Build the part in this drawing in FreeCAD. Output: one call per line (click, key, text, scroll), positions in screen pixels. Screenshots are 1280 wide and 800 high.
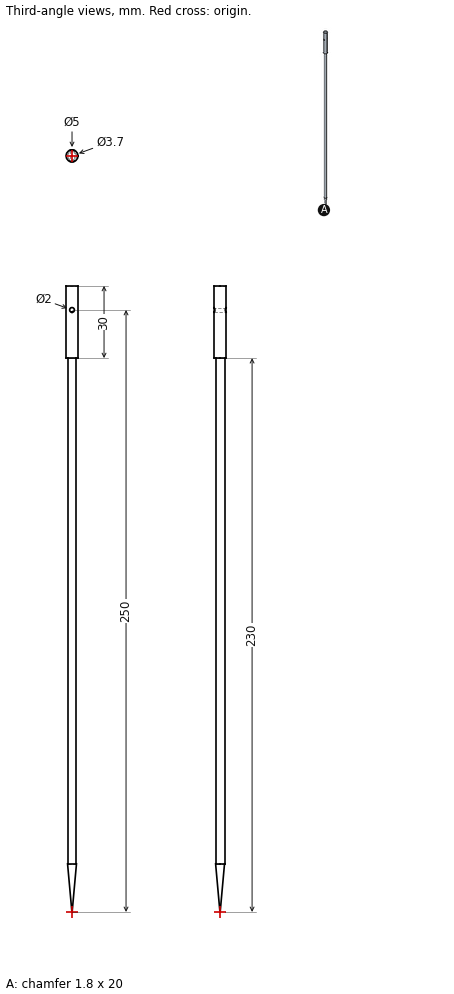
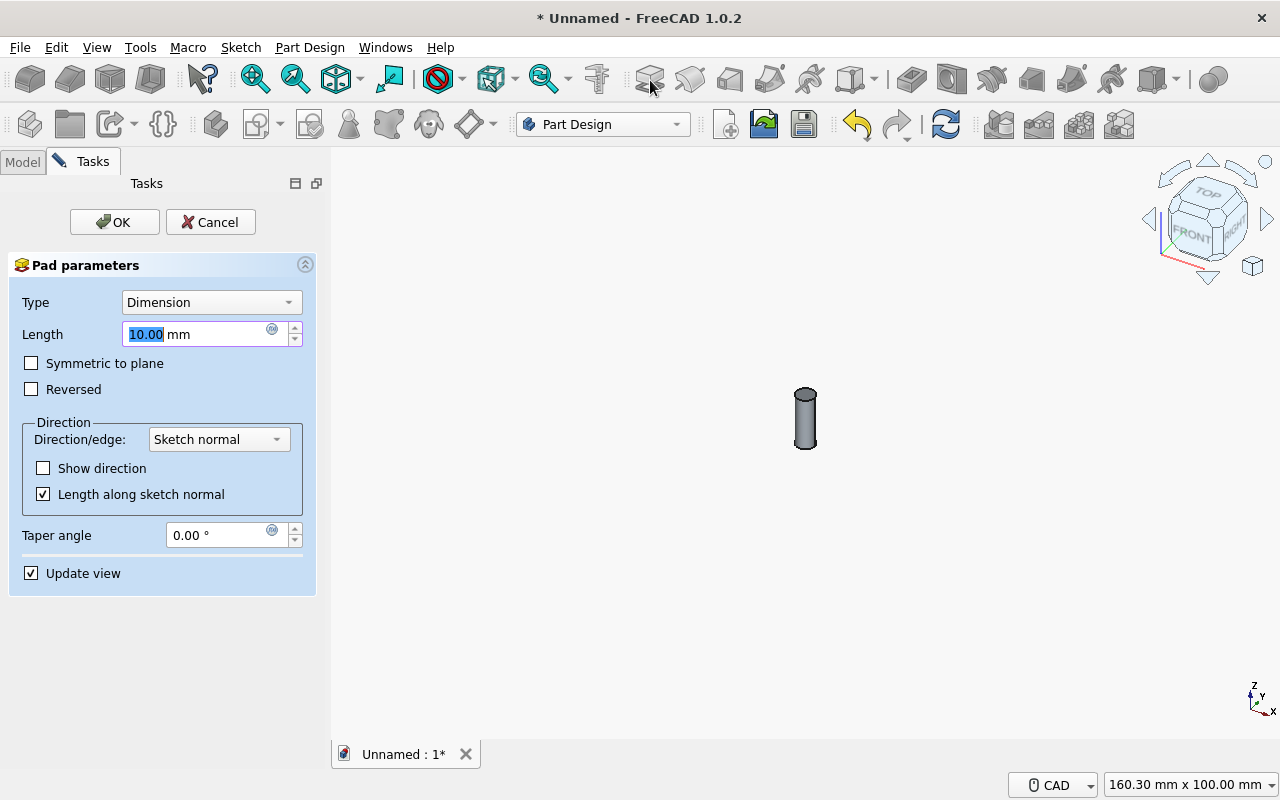
text(230)
key(Tab)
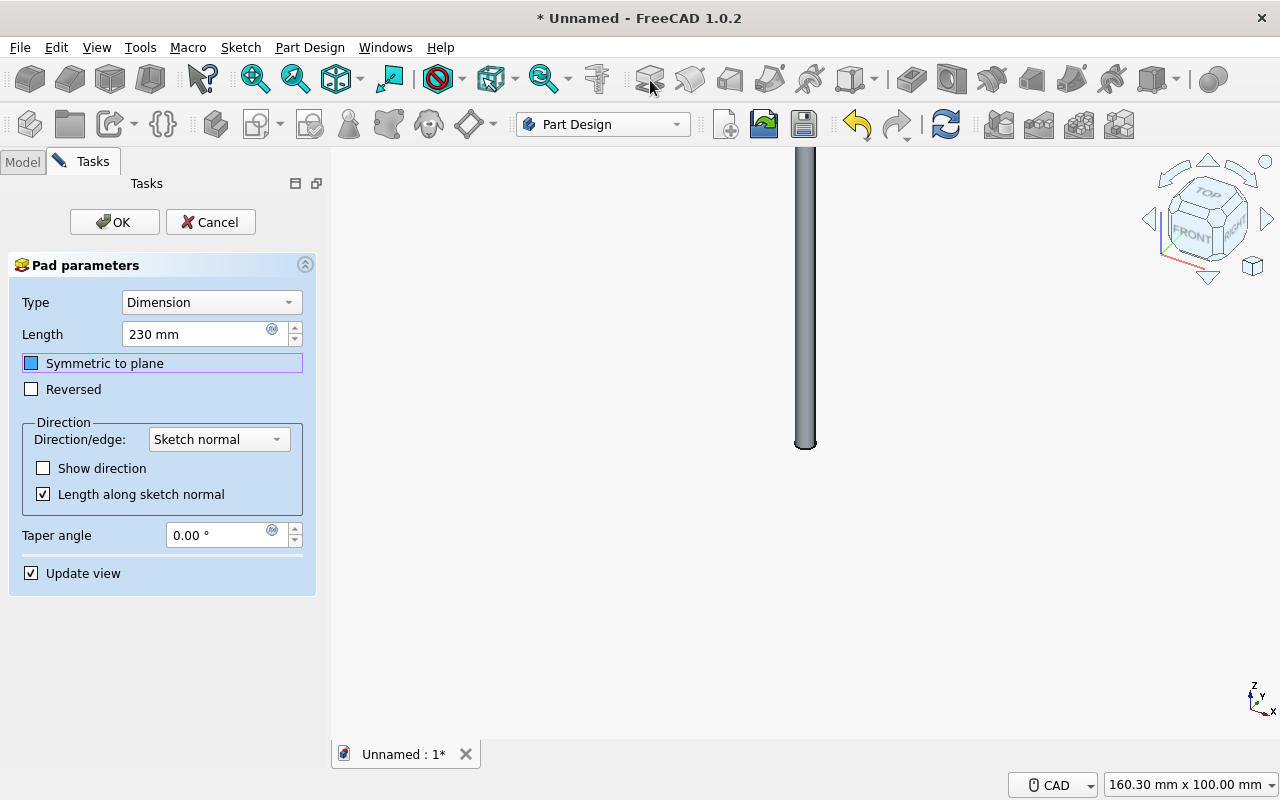
click(115, 222)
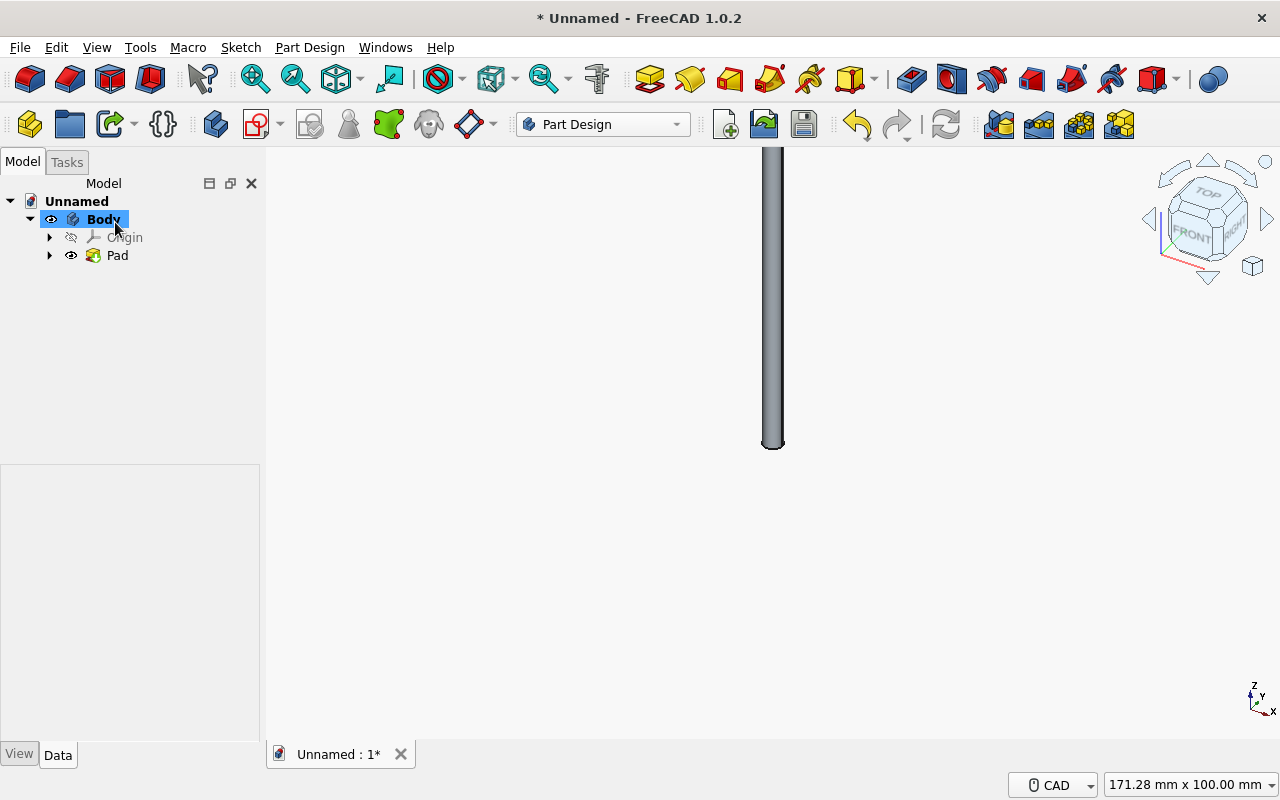
click(256, 80)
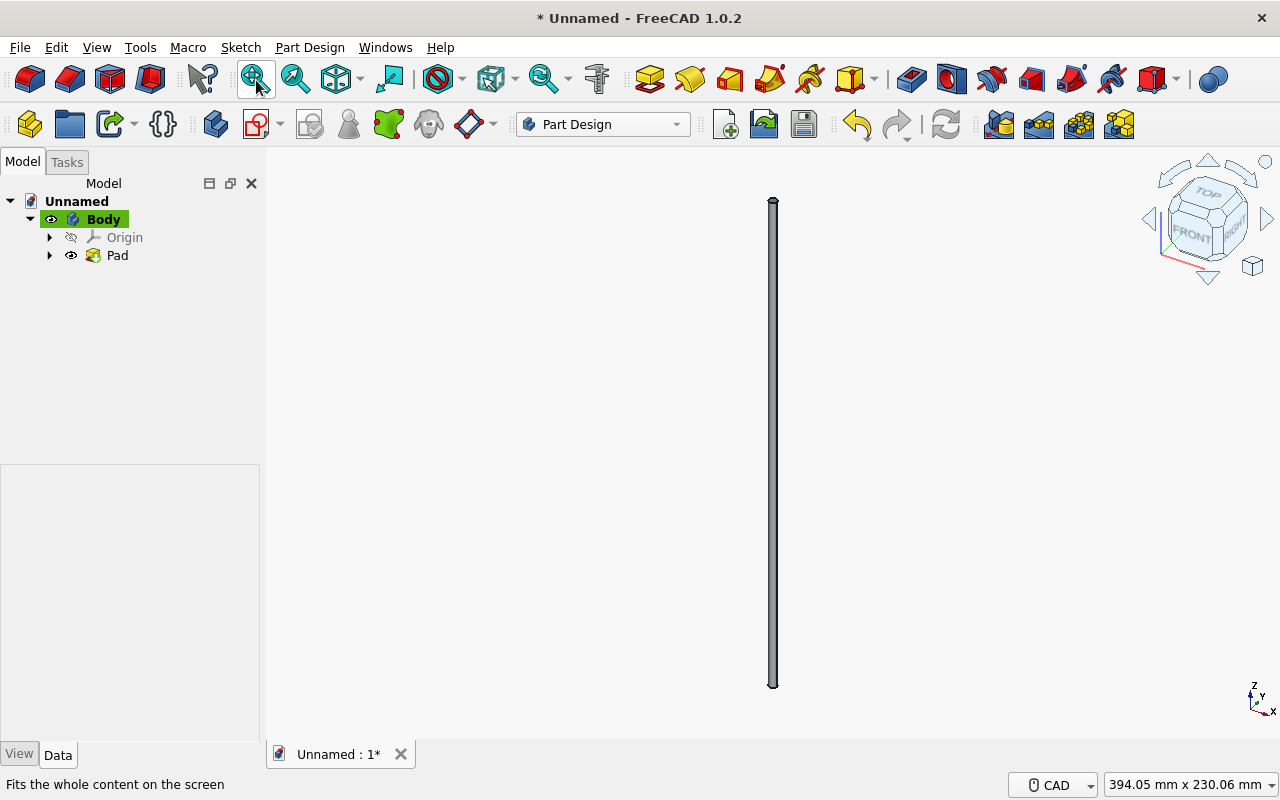
scroll(773, 200, up, 5)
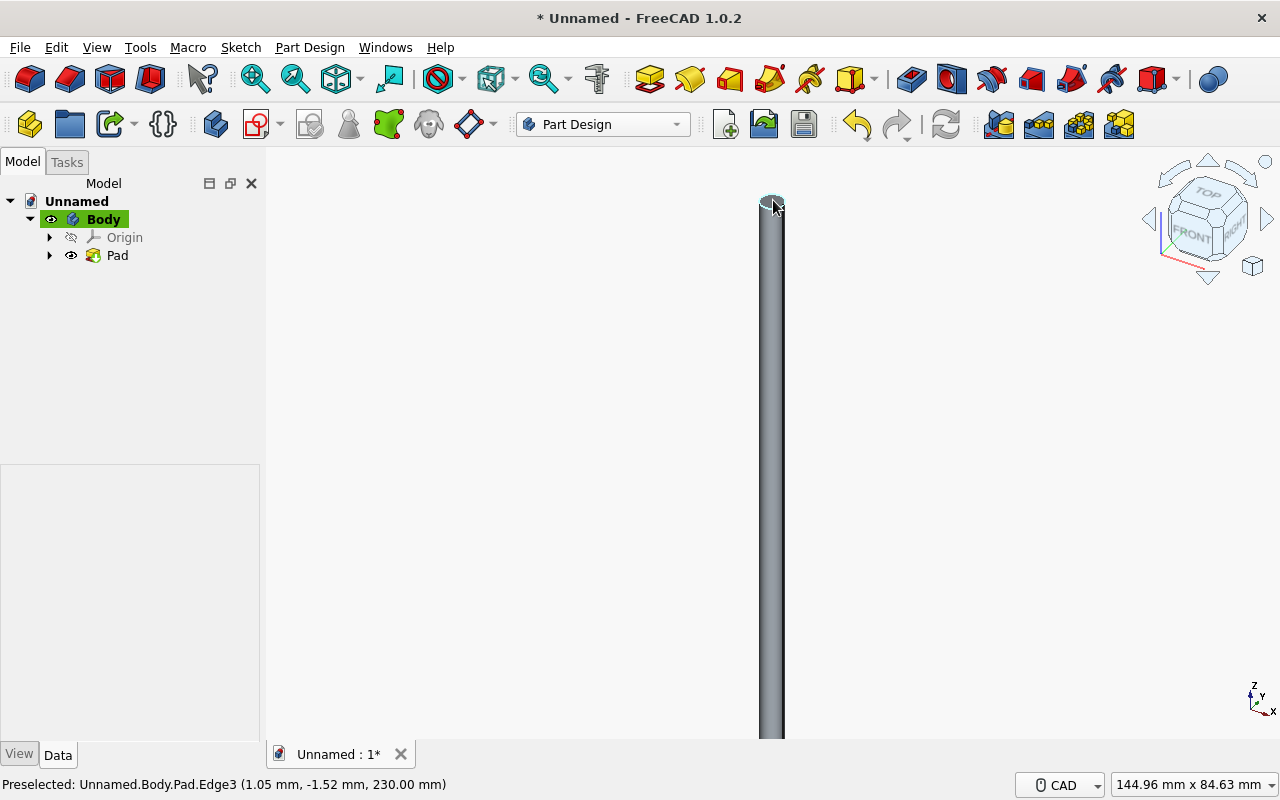
click(774, 199)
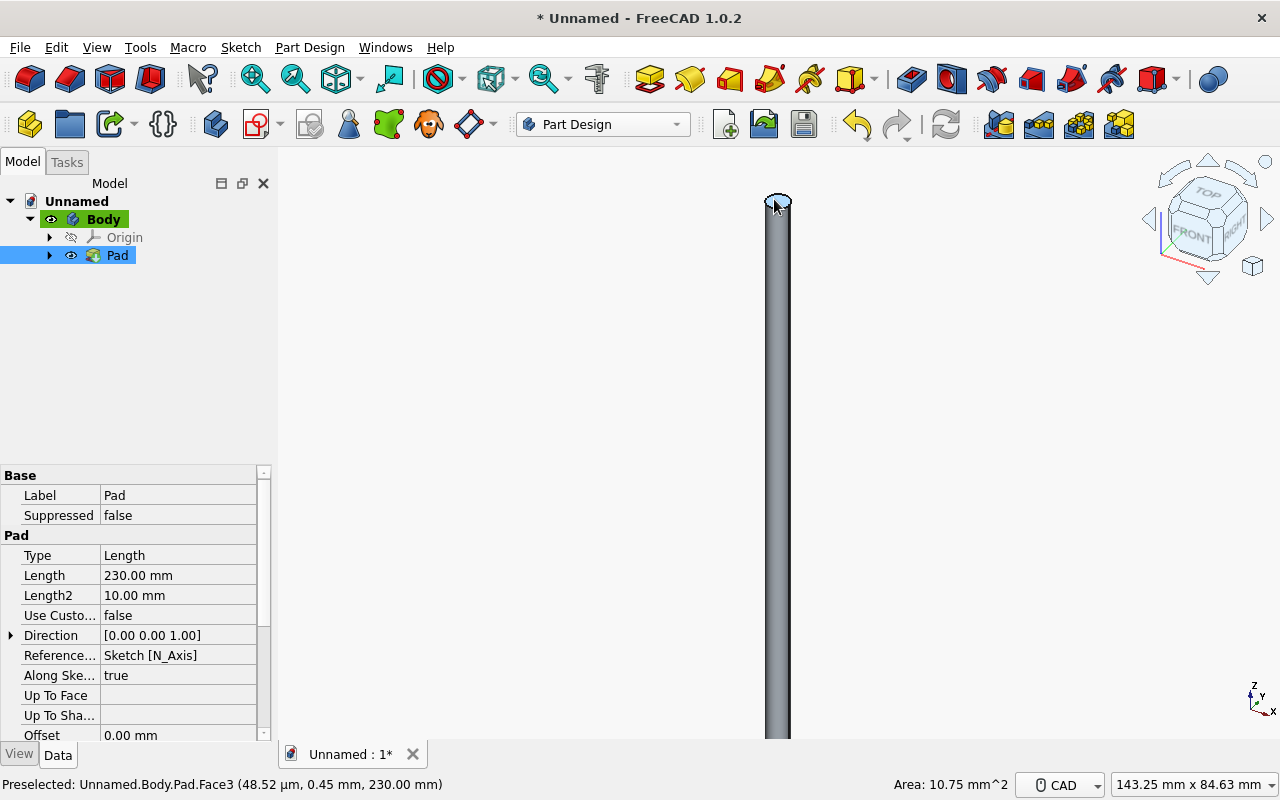
click(256, 124)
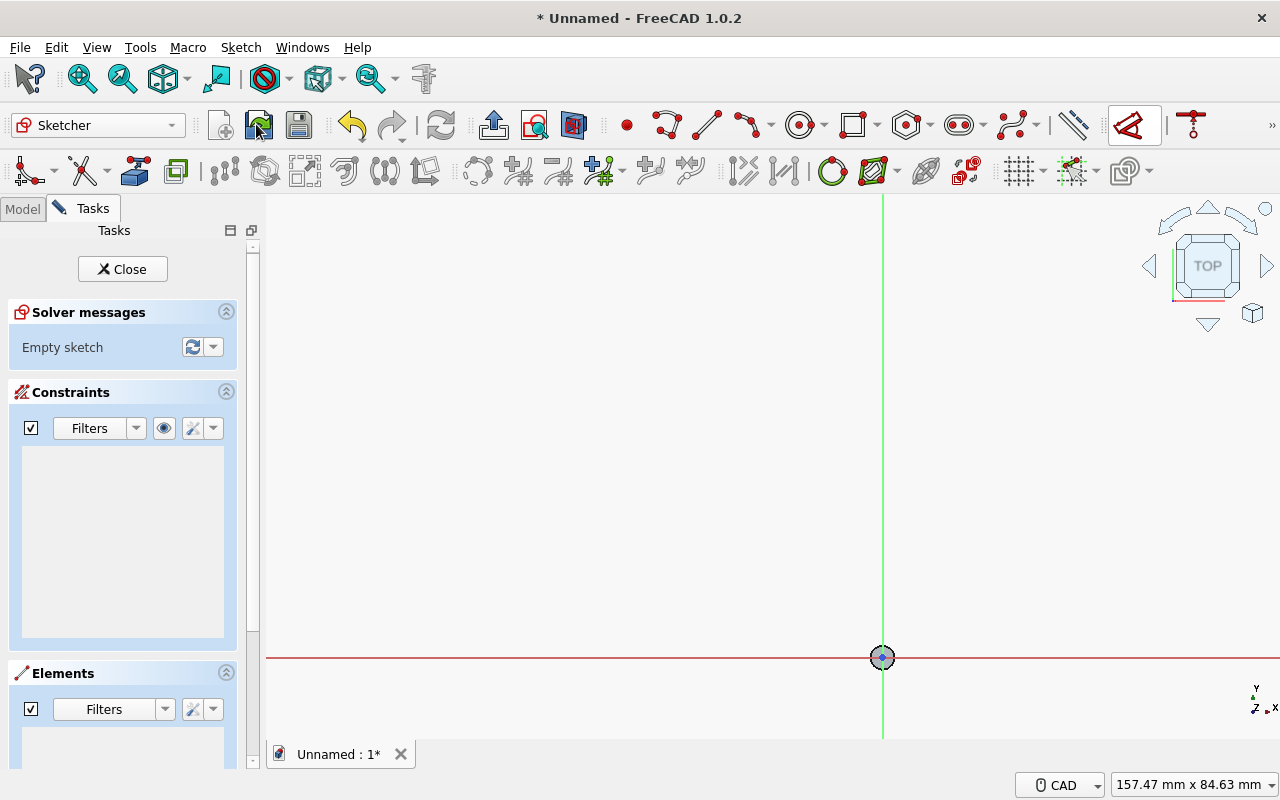
scroll(900, 677, up, 12)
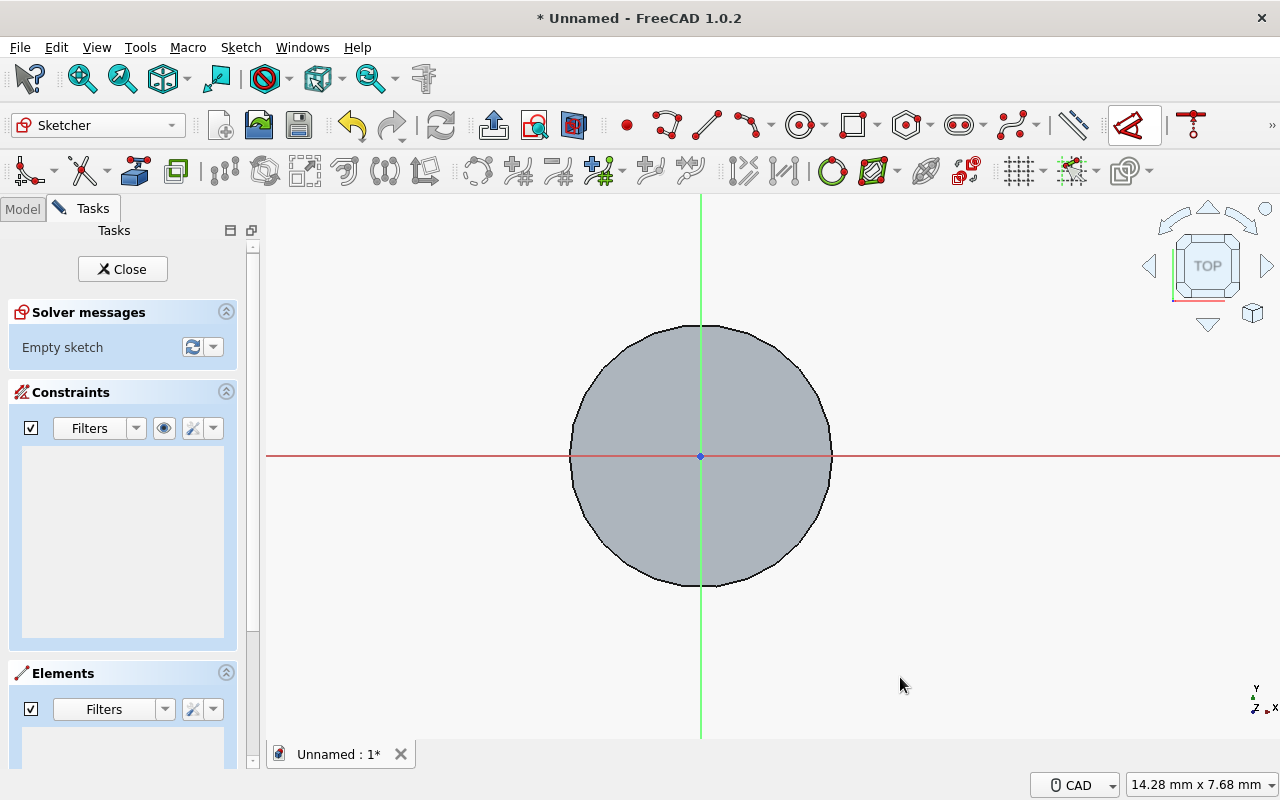
click(800, 126)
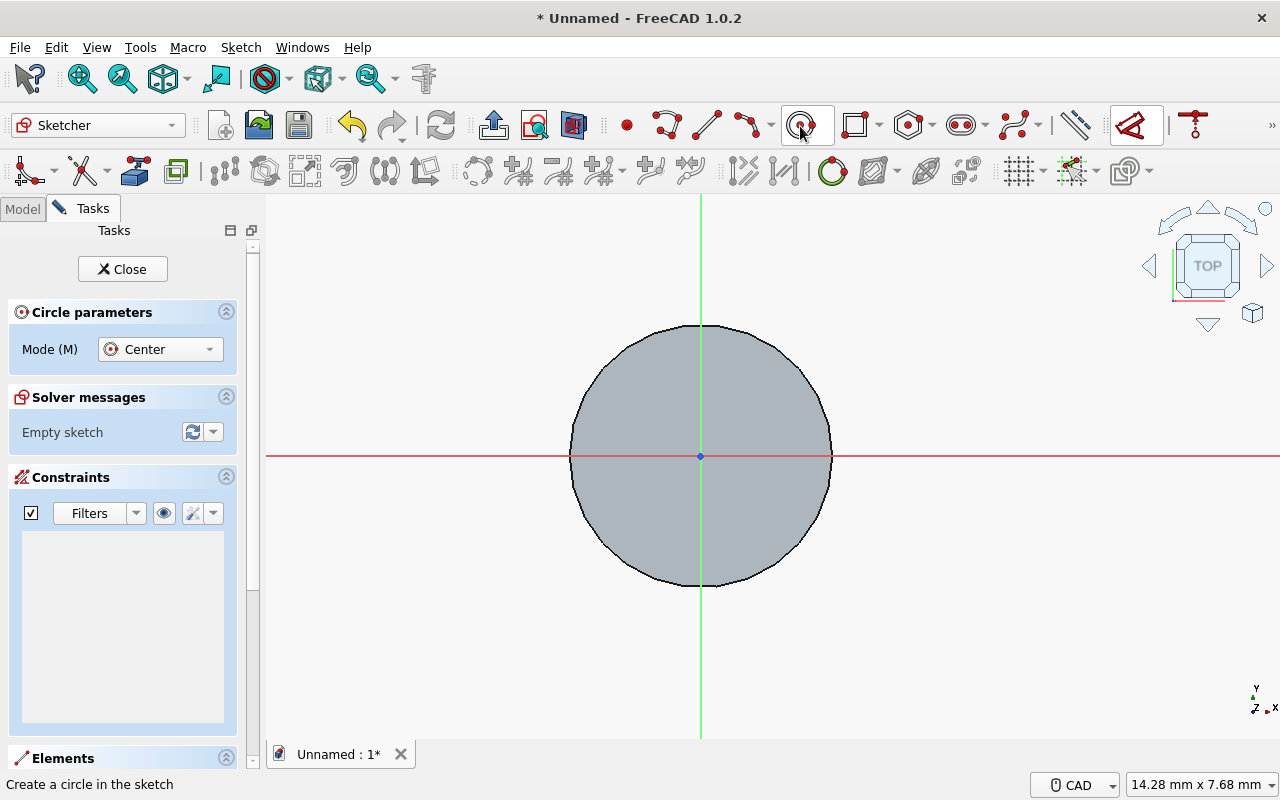
click(701, 456)
move(826, 331)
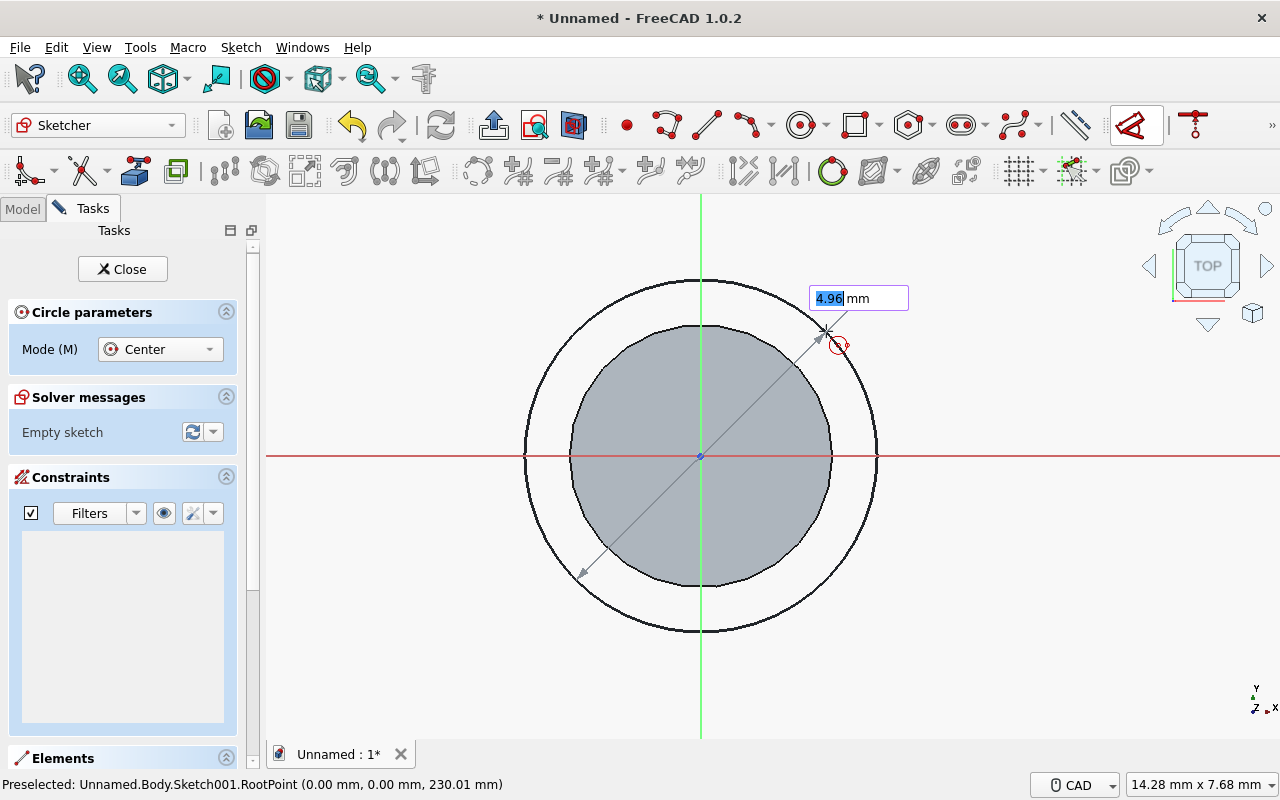
text(5)
key(Return)
key(Escape)